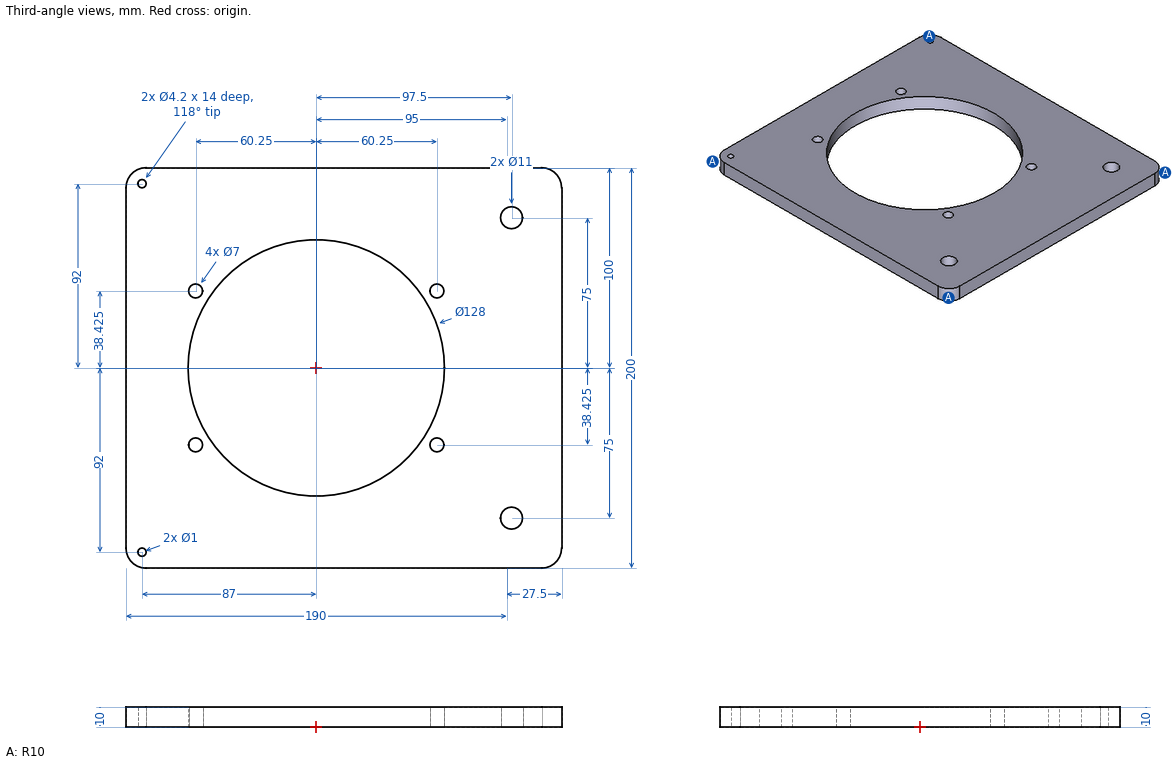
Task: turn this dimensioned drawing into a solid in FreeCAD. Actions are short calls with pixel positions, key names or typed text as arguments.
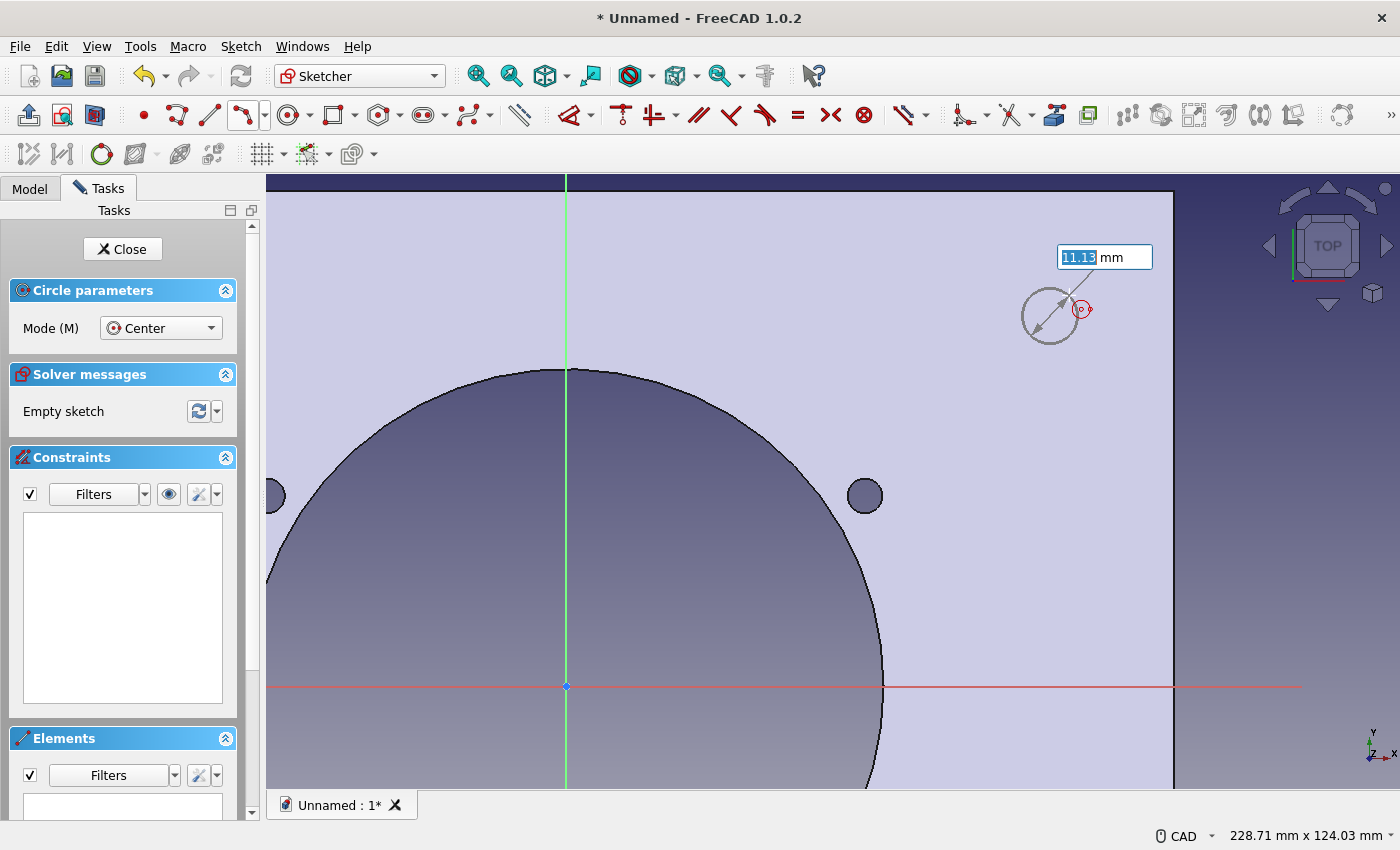
text(11)
key(Return)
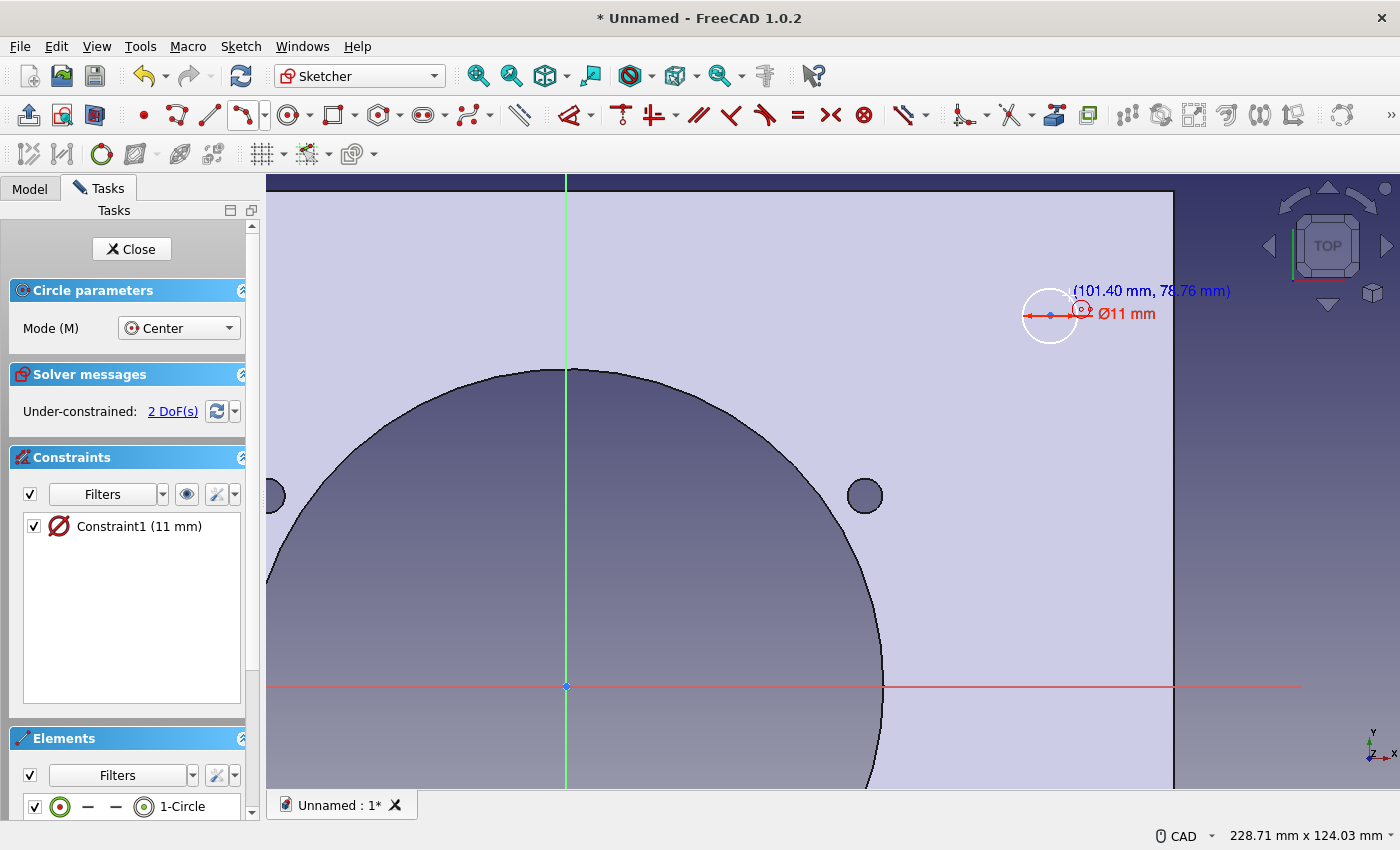
scroll(718, 314, down, 4)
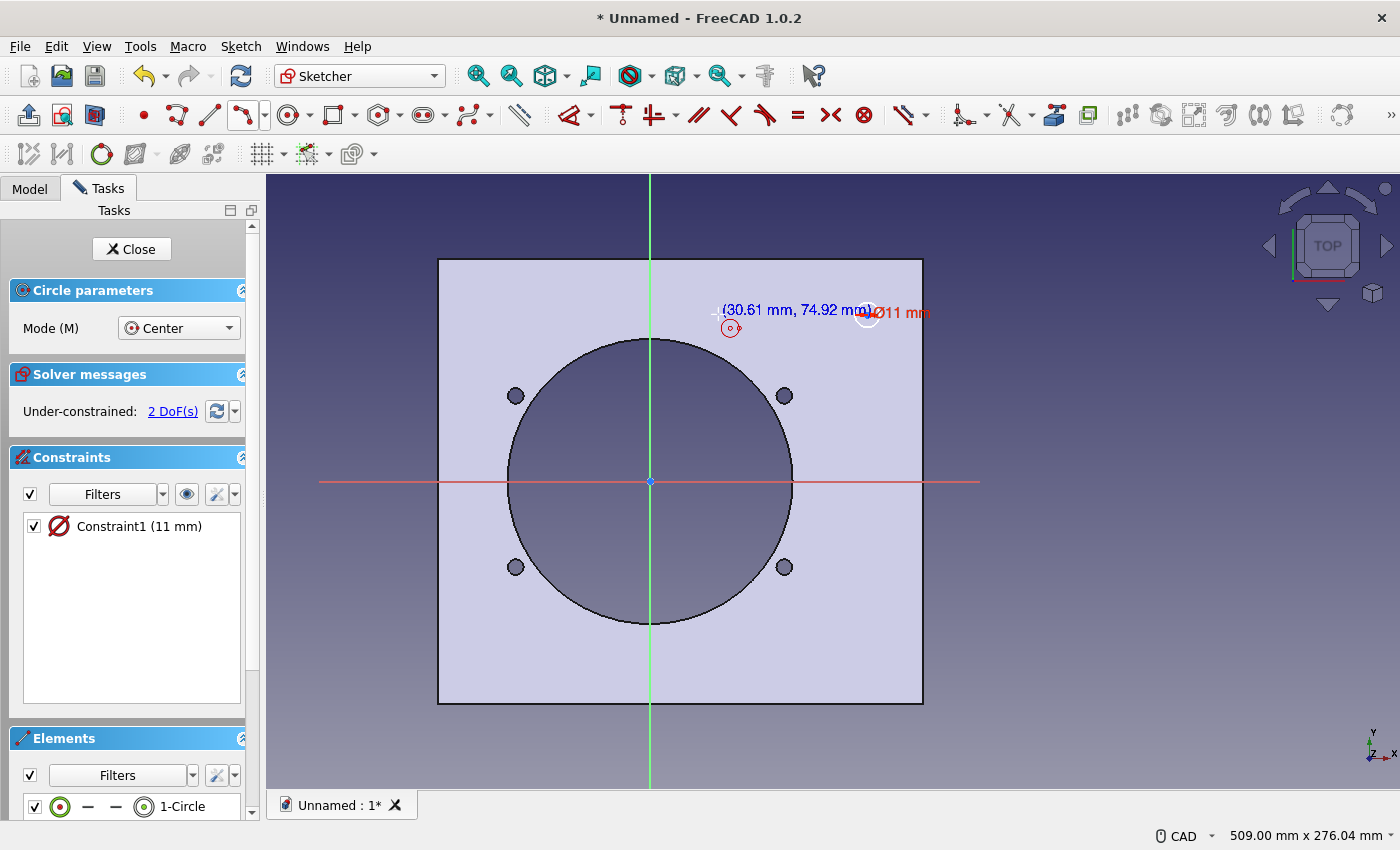
scroll(867, 649, up, 4)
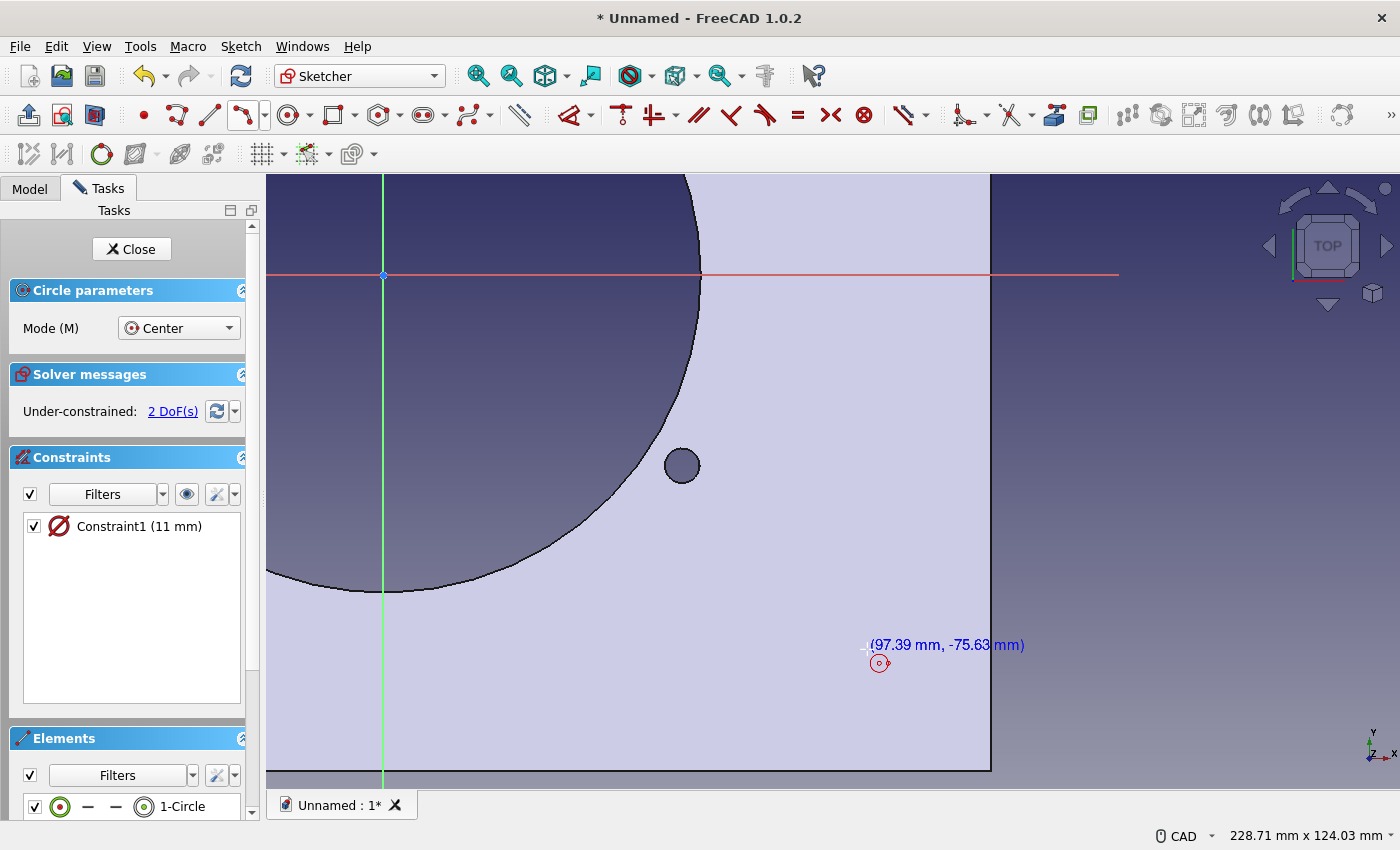
click(867, 647)
move(886, 628)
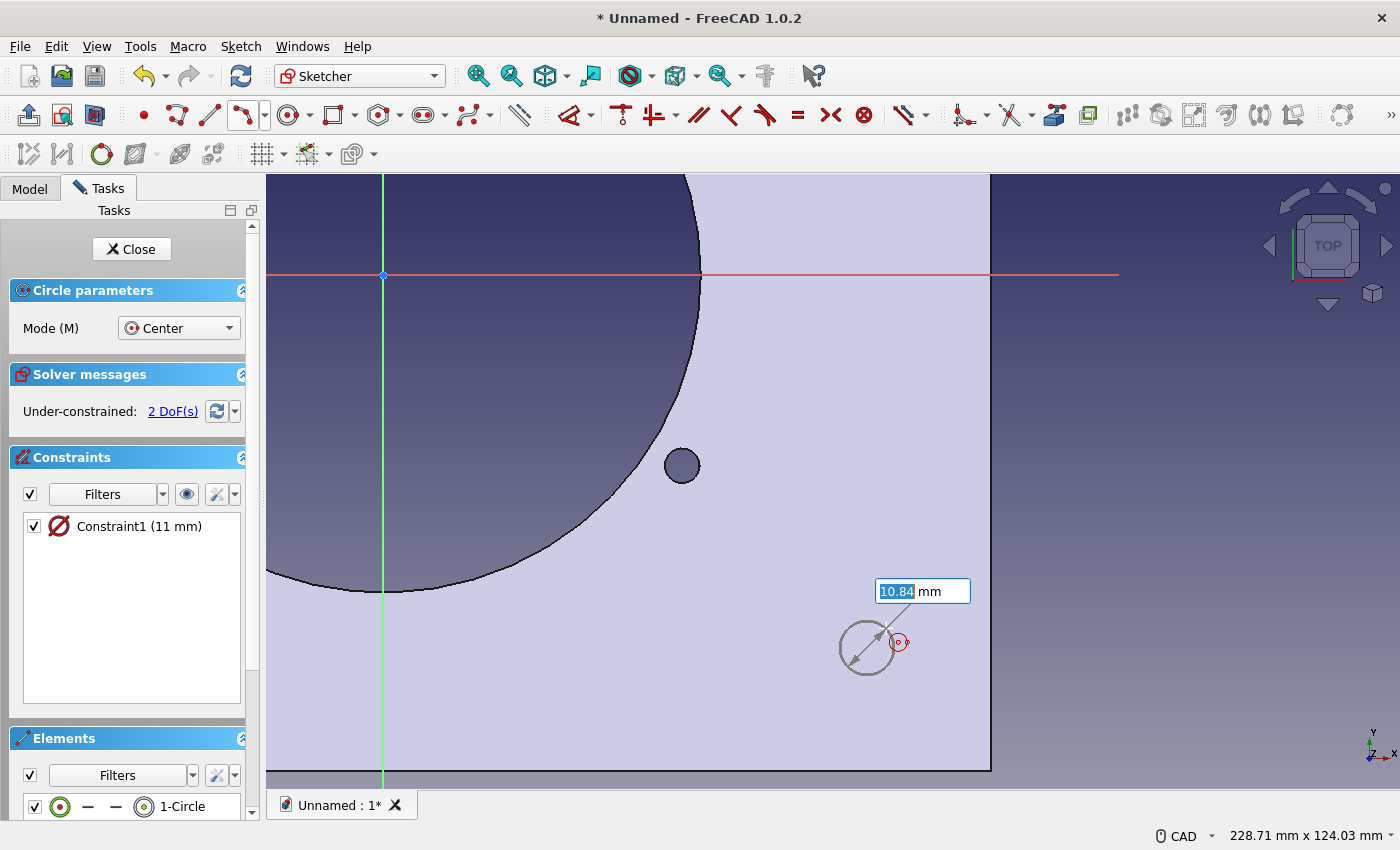
text(11)
key(Return)
key(Escape)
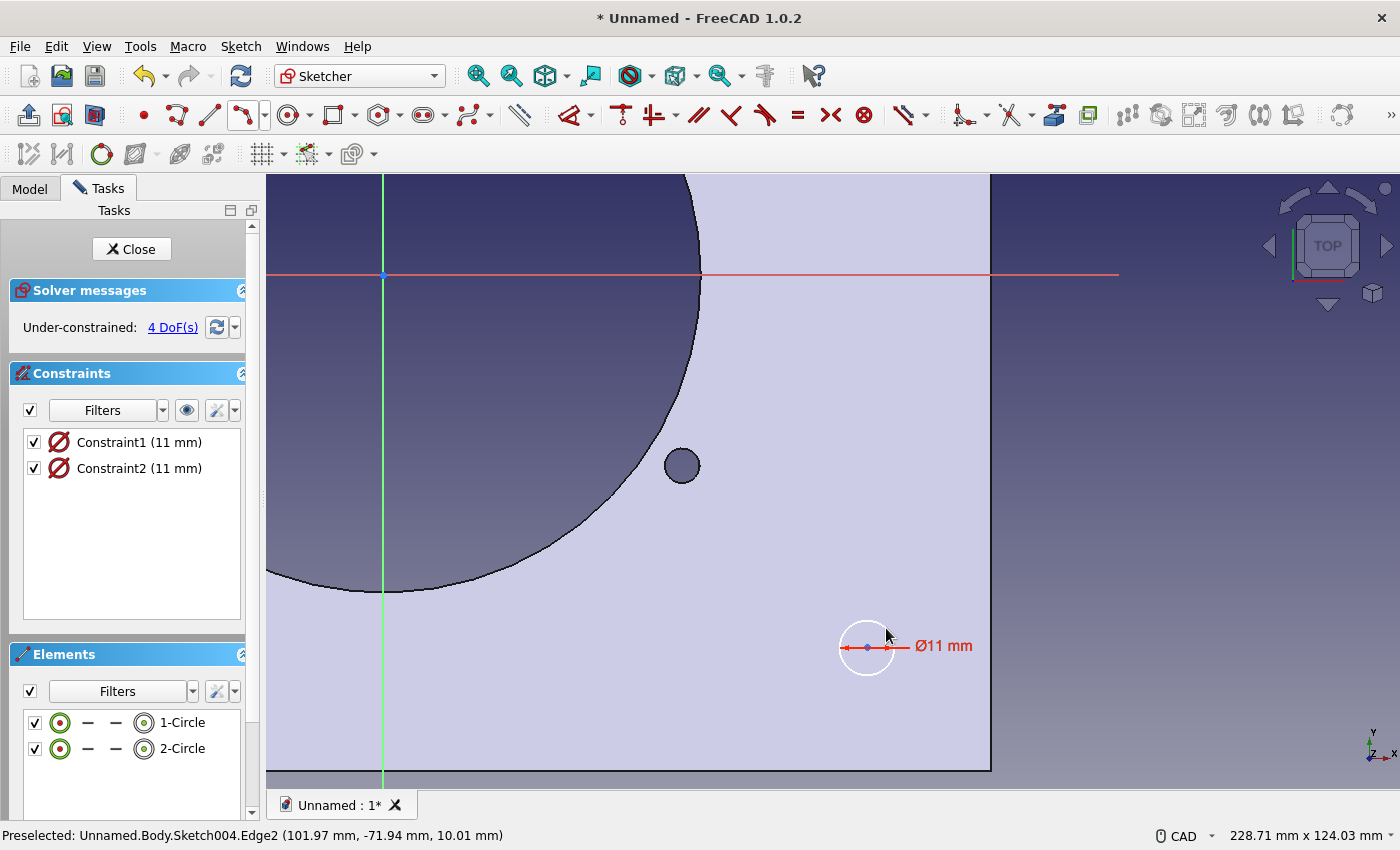
scroll(867, 650, down, 4)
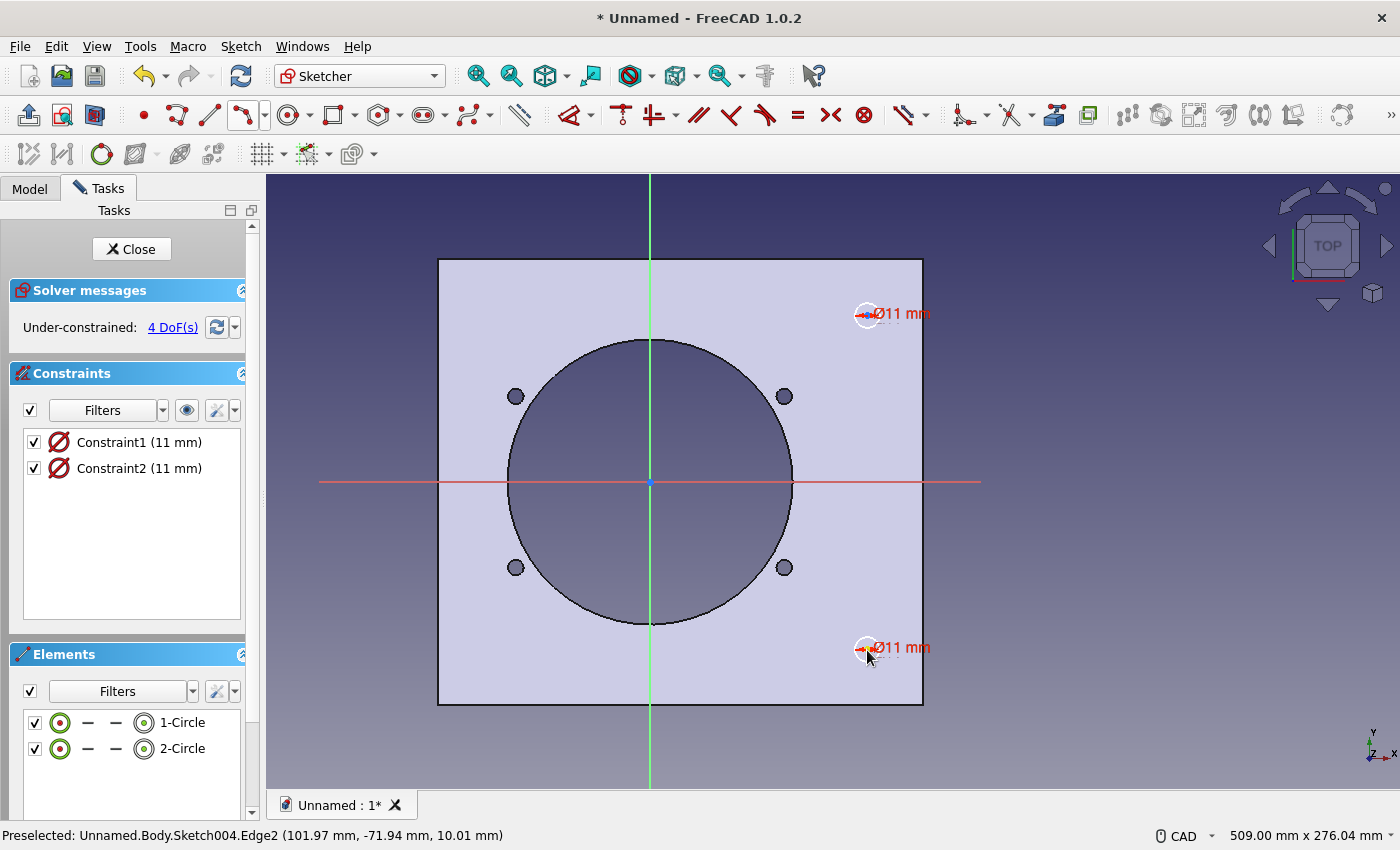
click(867, 316)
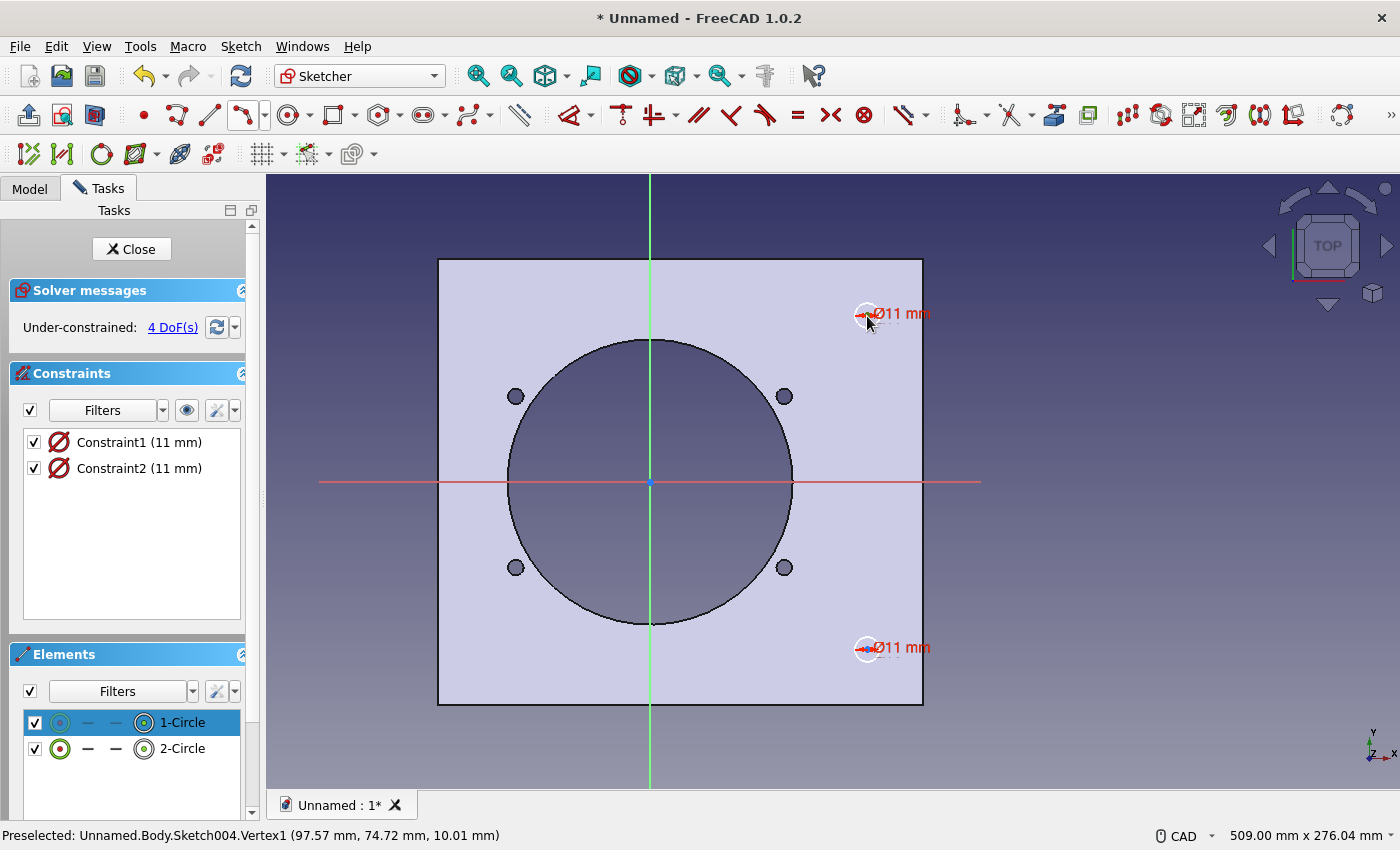
click(867, 650)